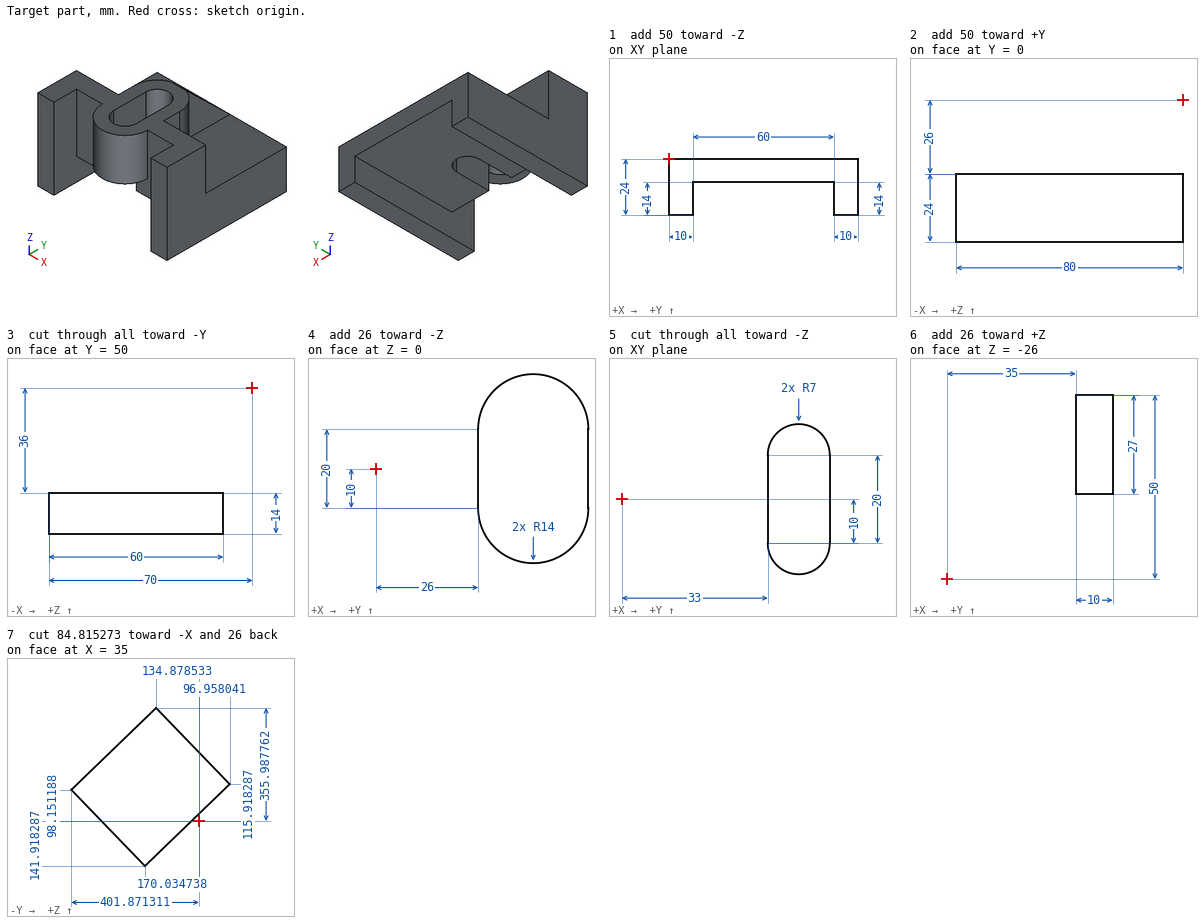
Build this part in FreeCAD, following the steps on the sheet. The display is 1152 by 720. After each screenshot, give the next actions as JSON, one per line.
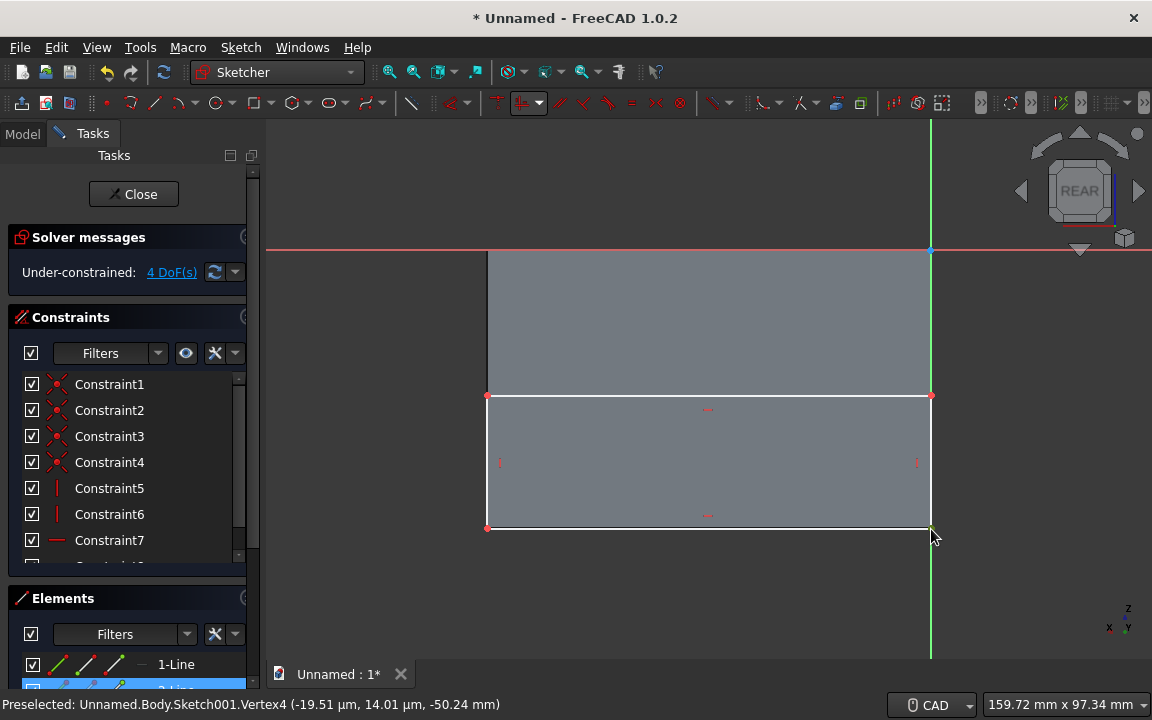
{"action": "left_click", "coordinate": [931, 596]}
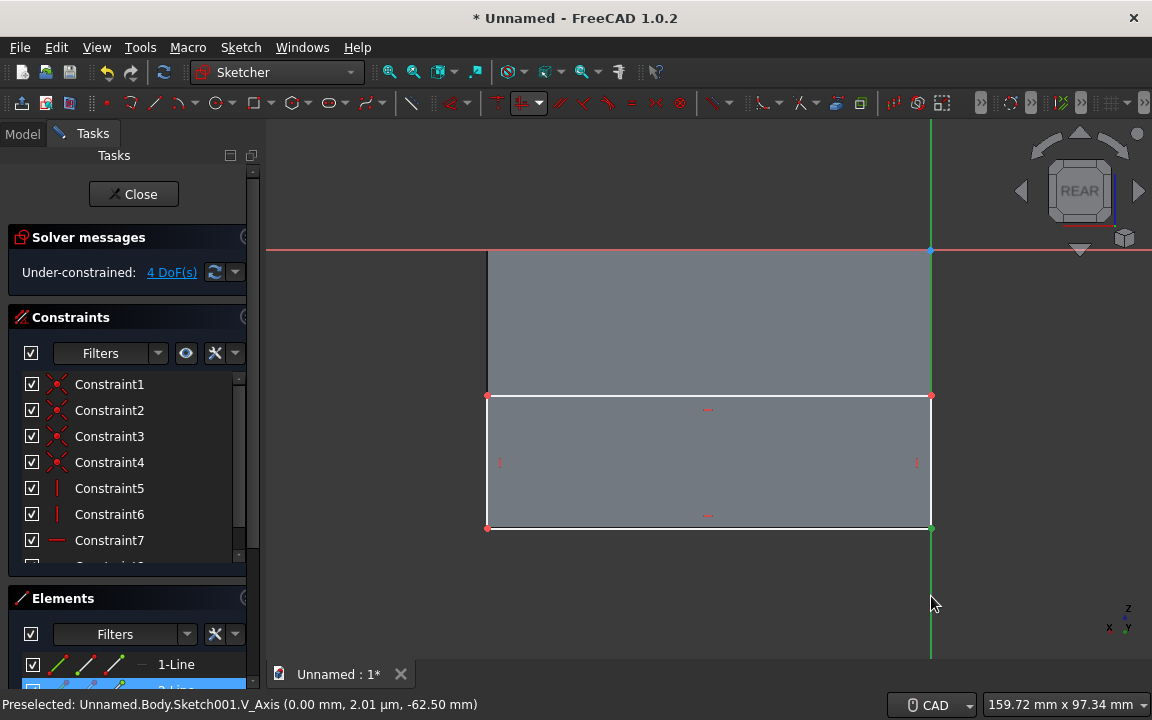
{"action": "key", "text": "c"}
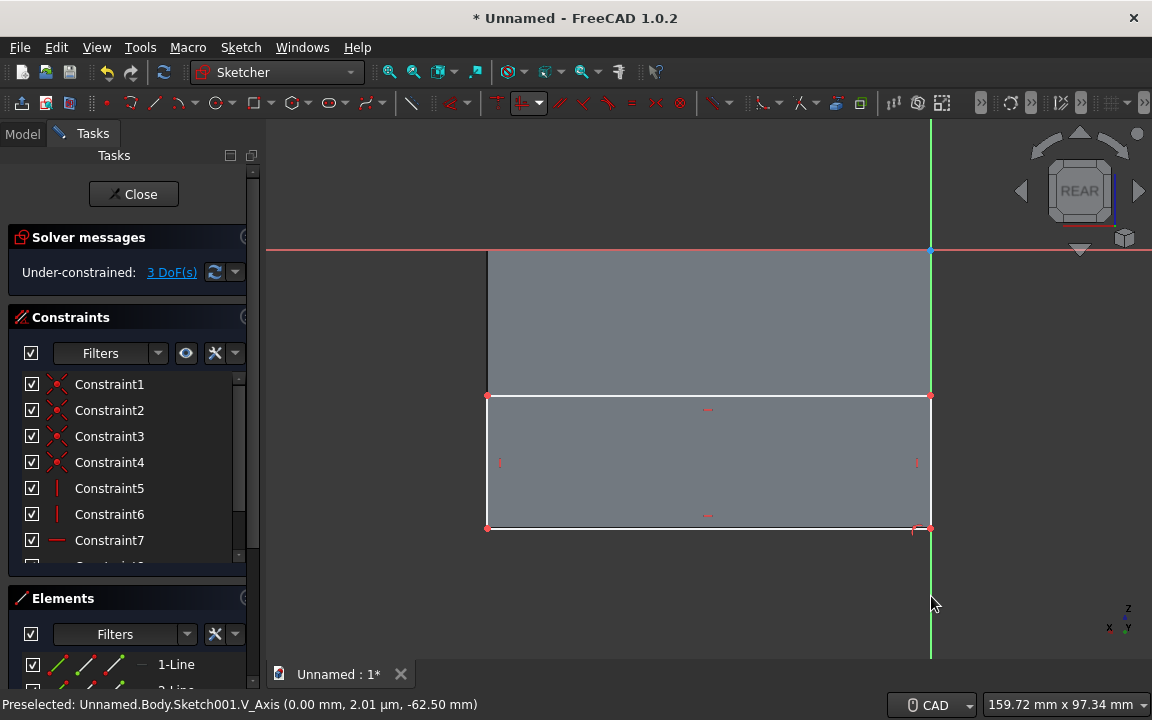
{"action": "key", "text": "d"}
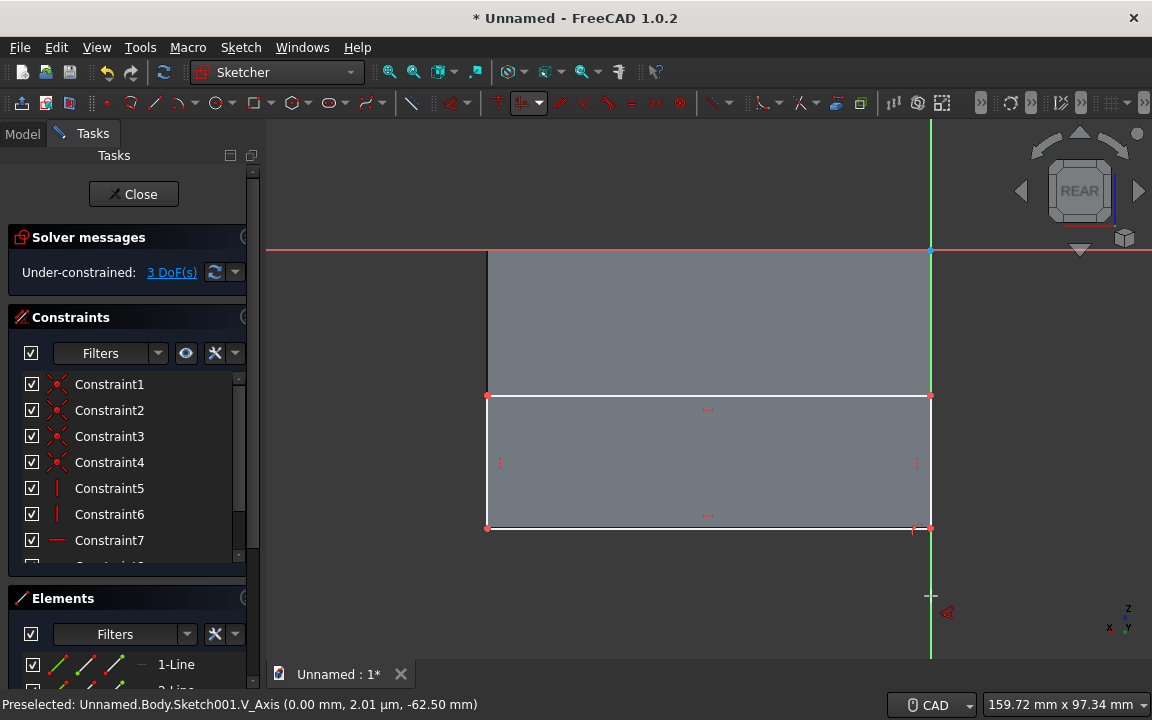
{"action": "left_click", "coordinate": [487, 436]}
{"action": "left_click", "coordinate": [453, 462]}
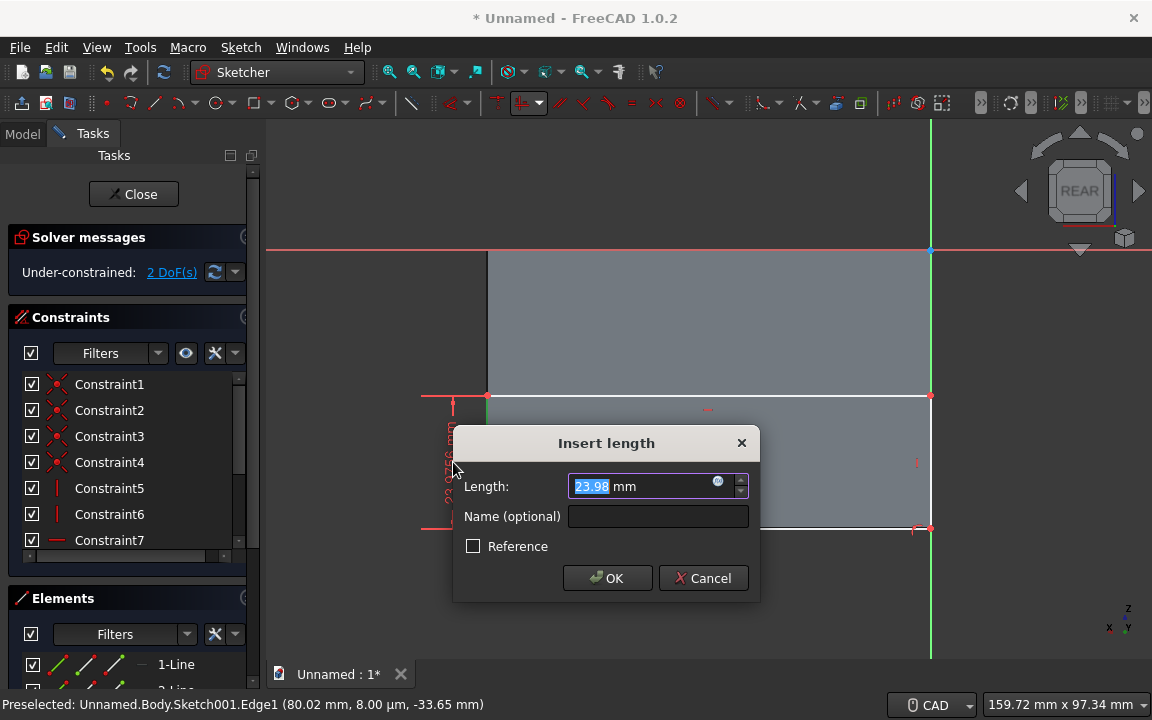
{"action": "type", "text": "24"}
{"action": "key", "text": "Return"}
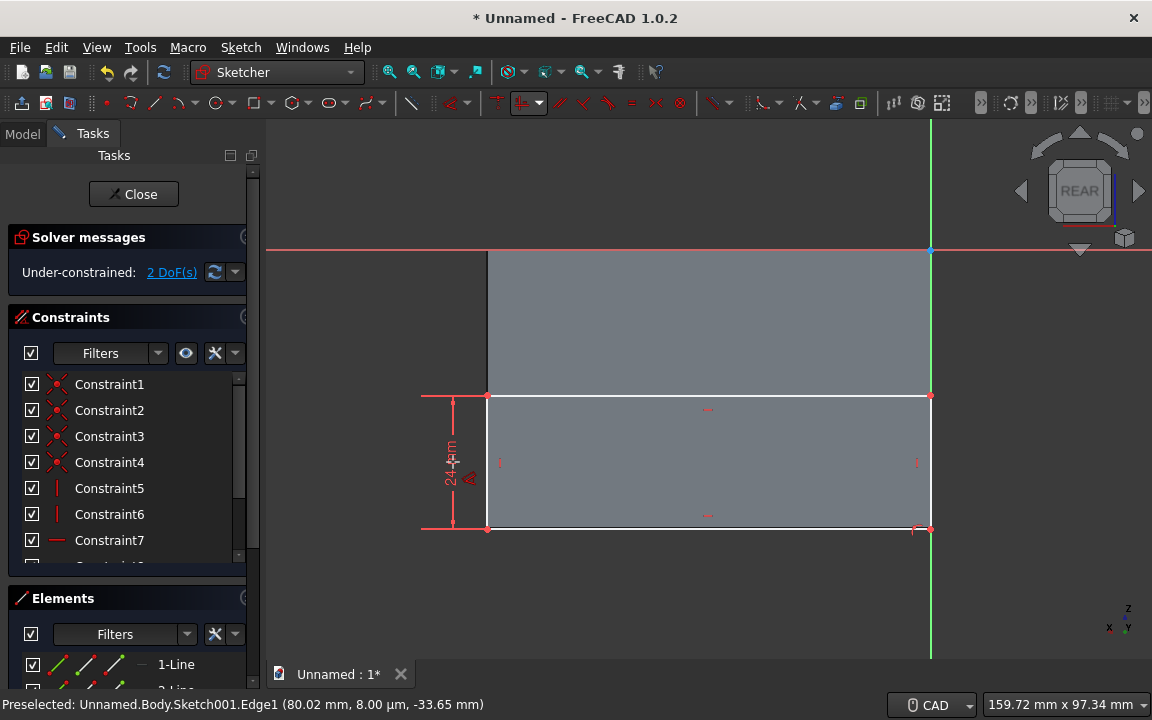
{"action": "left_click", "coordinate": [620, 529]}
{"action": "left_click", "coordinate": [709, 563]}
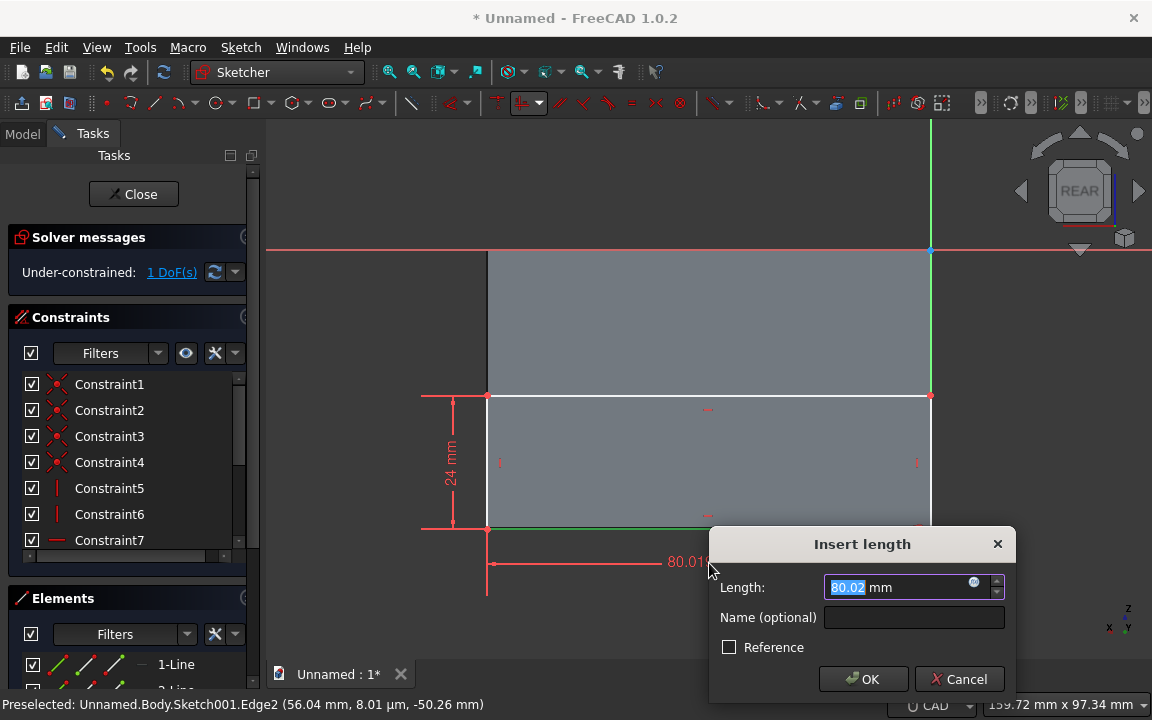
{"action": "type", "text": "80"}
{"action": "key", "text": "Return"}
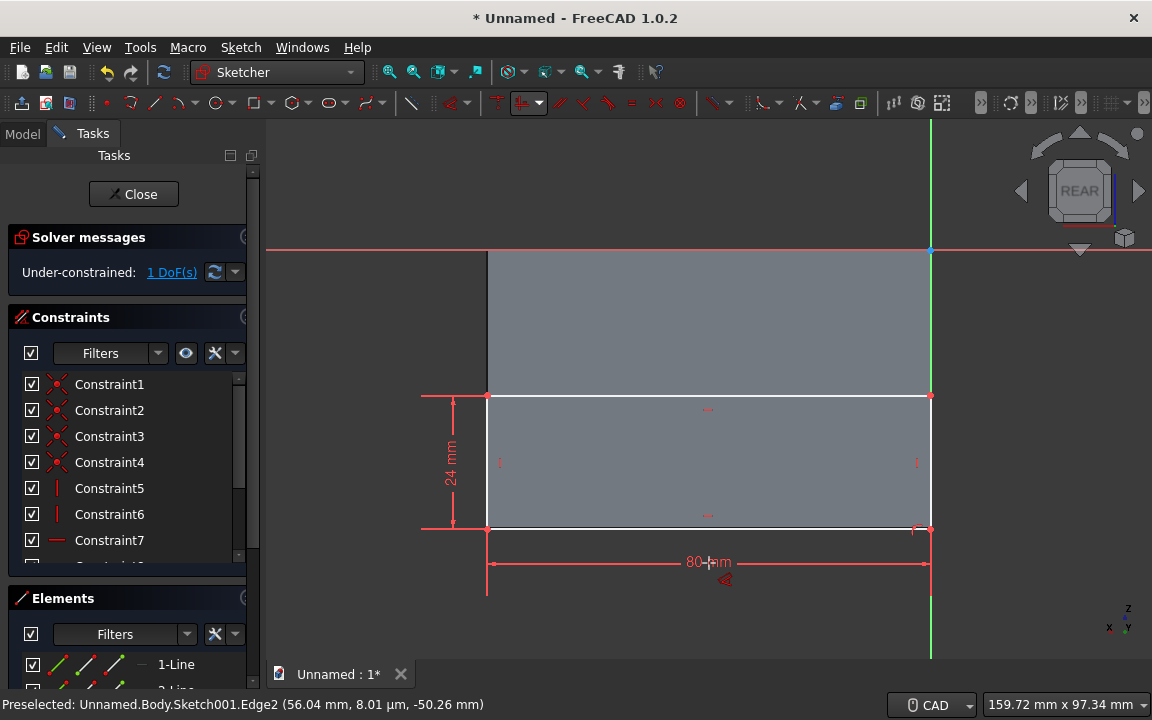
{"action": "left_click", "coordinate": [487, 396]}
{"action": "left_click", "coordinate": [965, 323]}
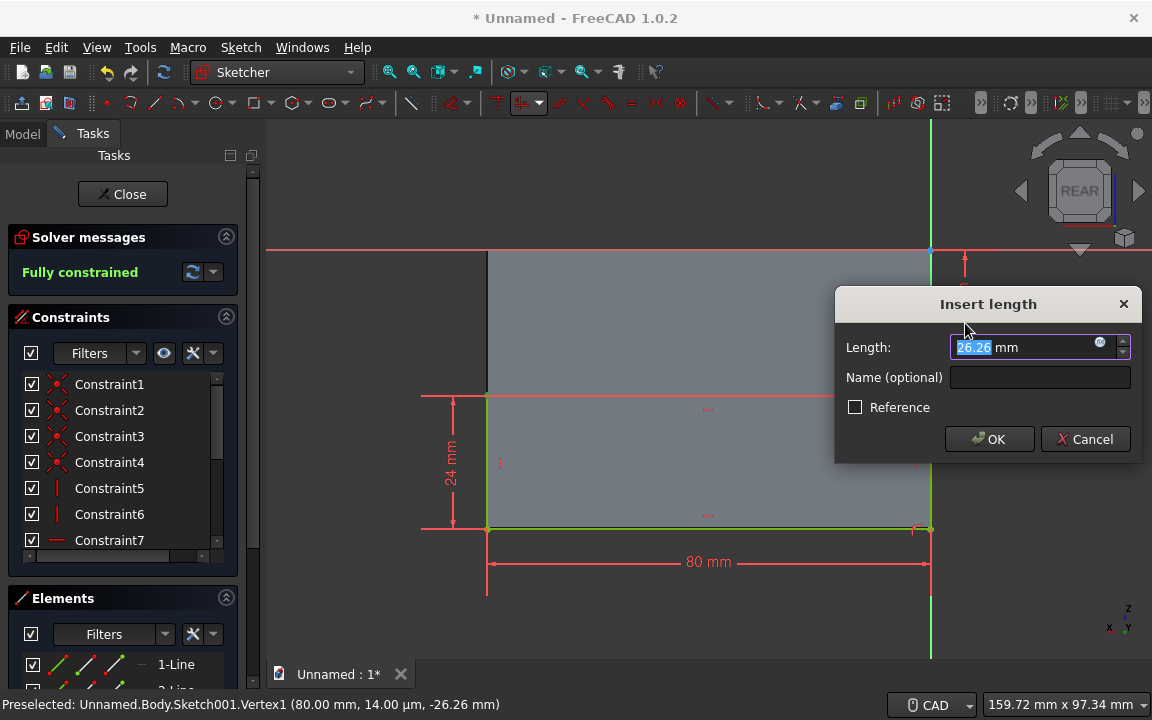
{"action": "type", "text": "26"}
{"action": "key", "text": "Return"}
{"action": "key", "text": "Escape"}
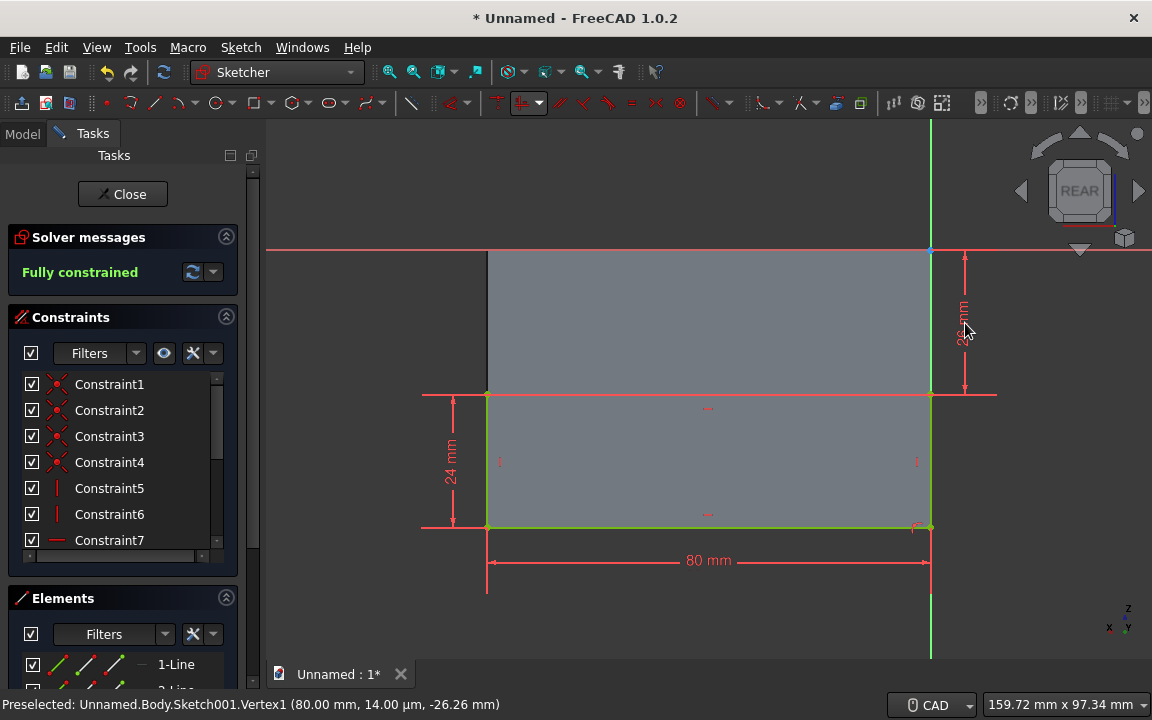
{"action": "left_click", "coordinate": [123, 194]}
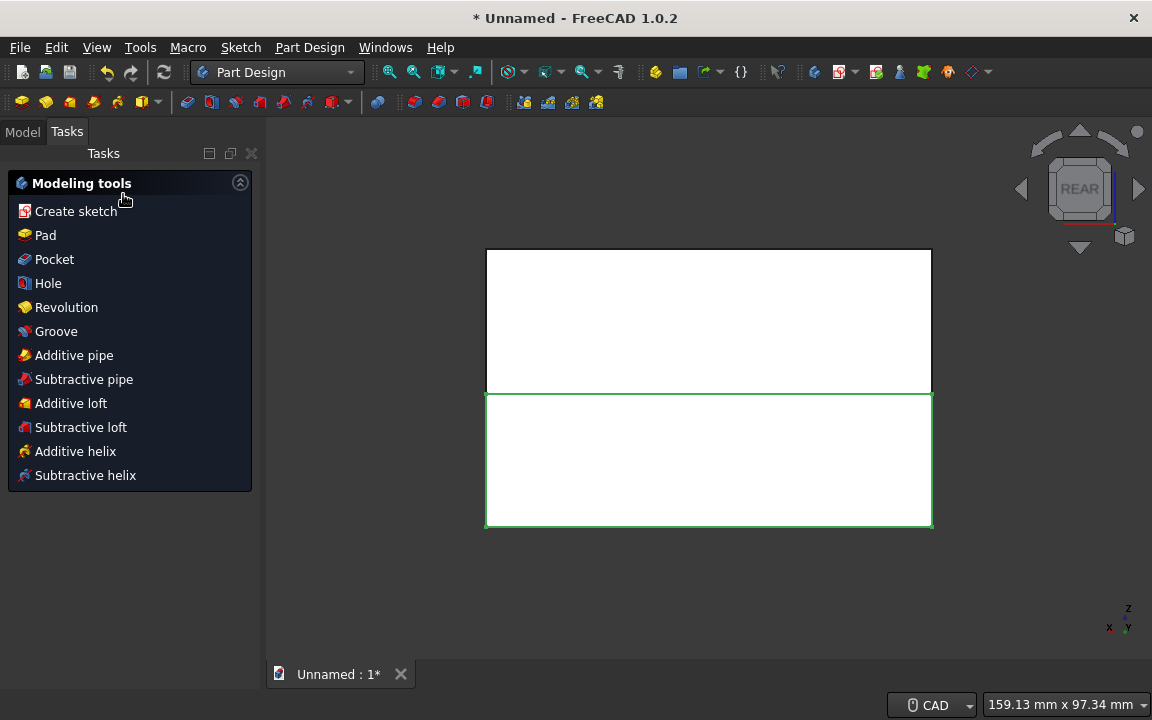
{"action": "left_click", "coordinate": [22, 102]}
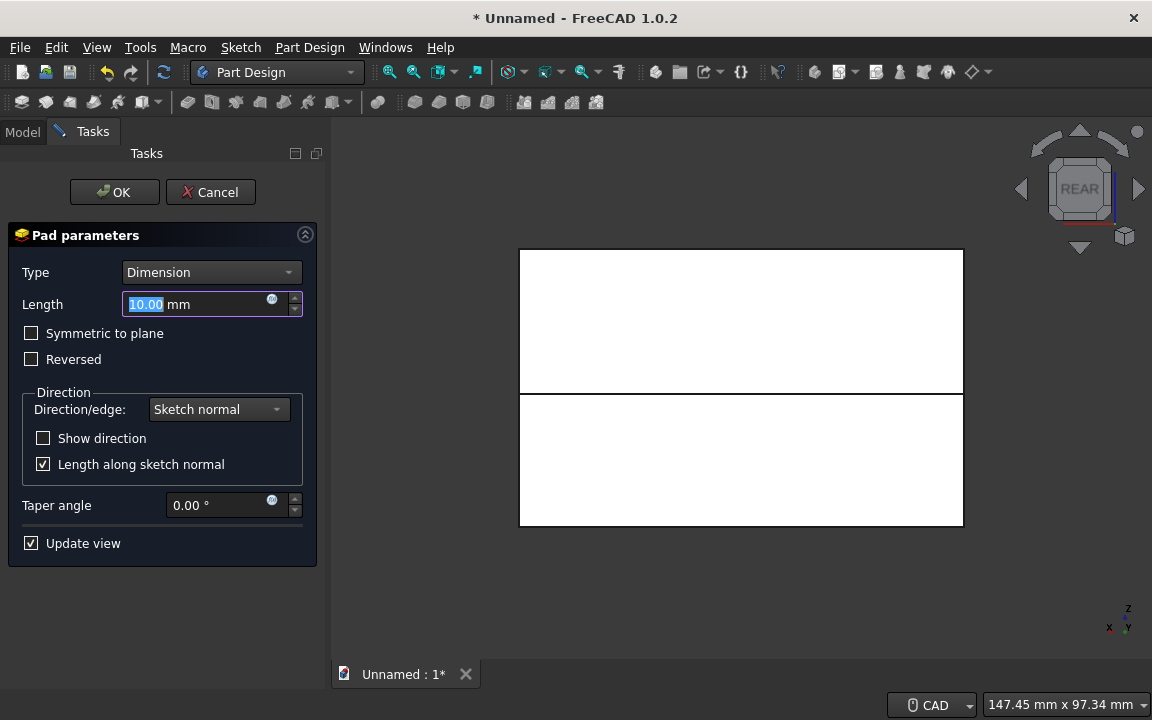
{"action": "type", "text": "50"}
{"action": "key", "text": "Tab"}